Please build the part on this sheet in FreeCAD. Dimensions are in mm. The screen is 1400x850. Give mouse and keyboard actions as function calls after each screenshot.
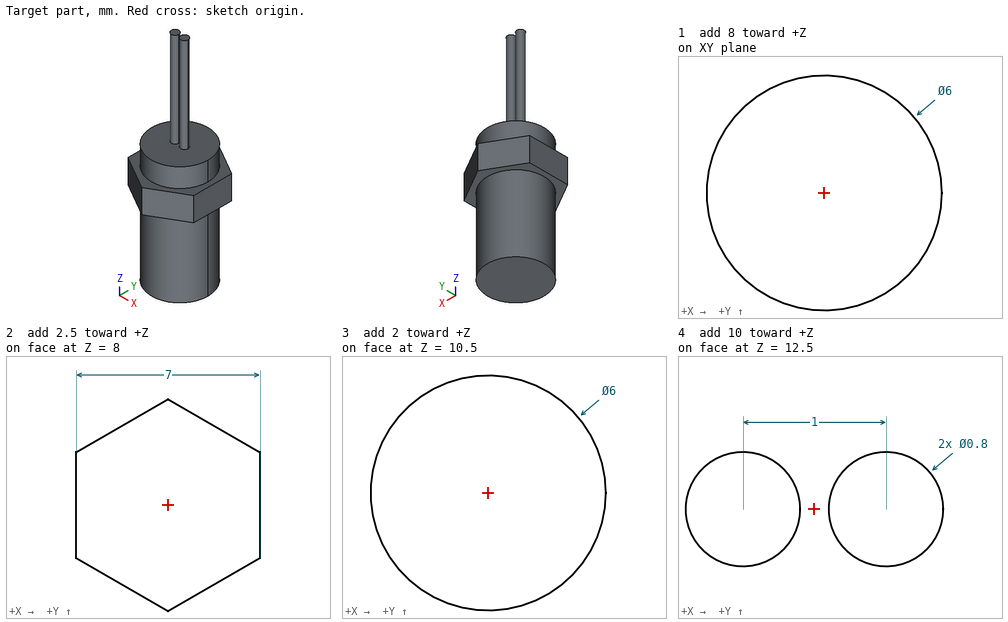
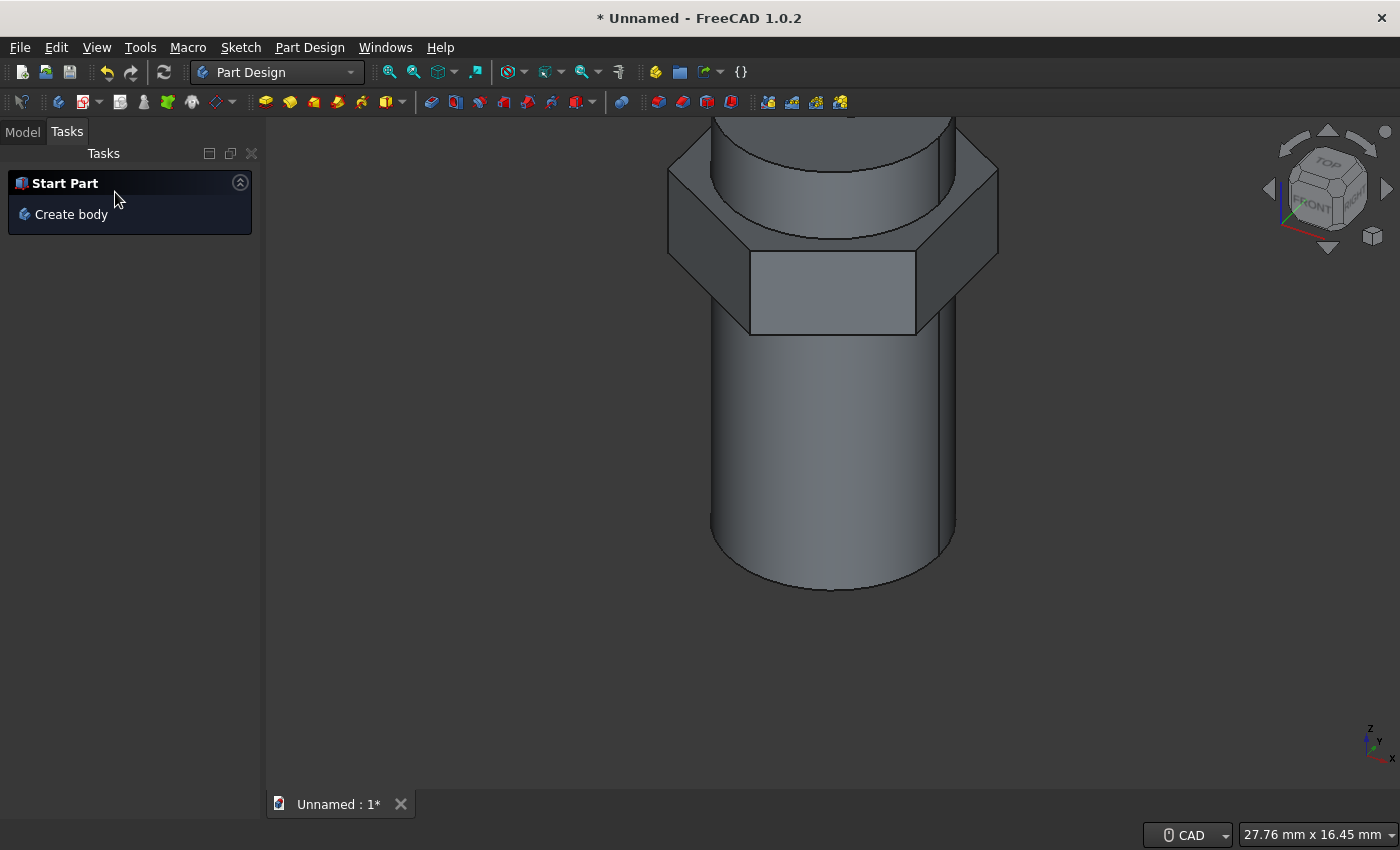
key(0)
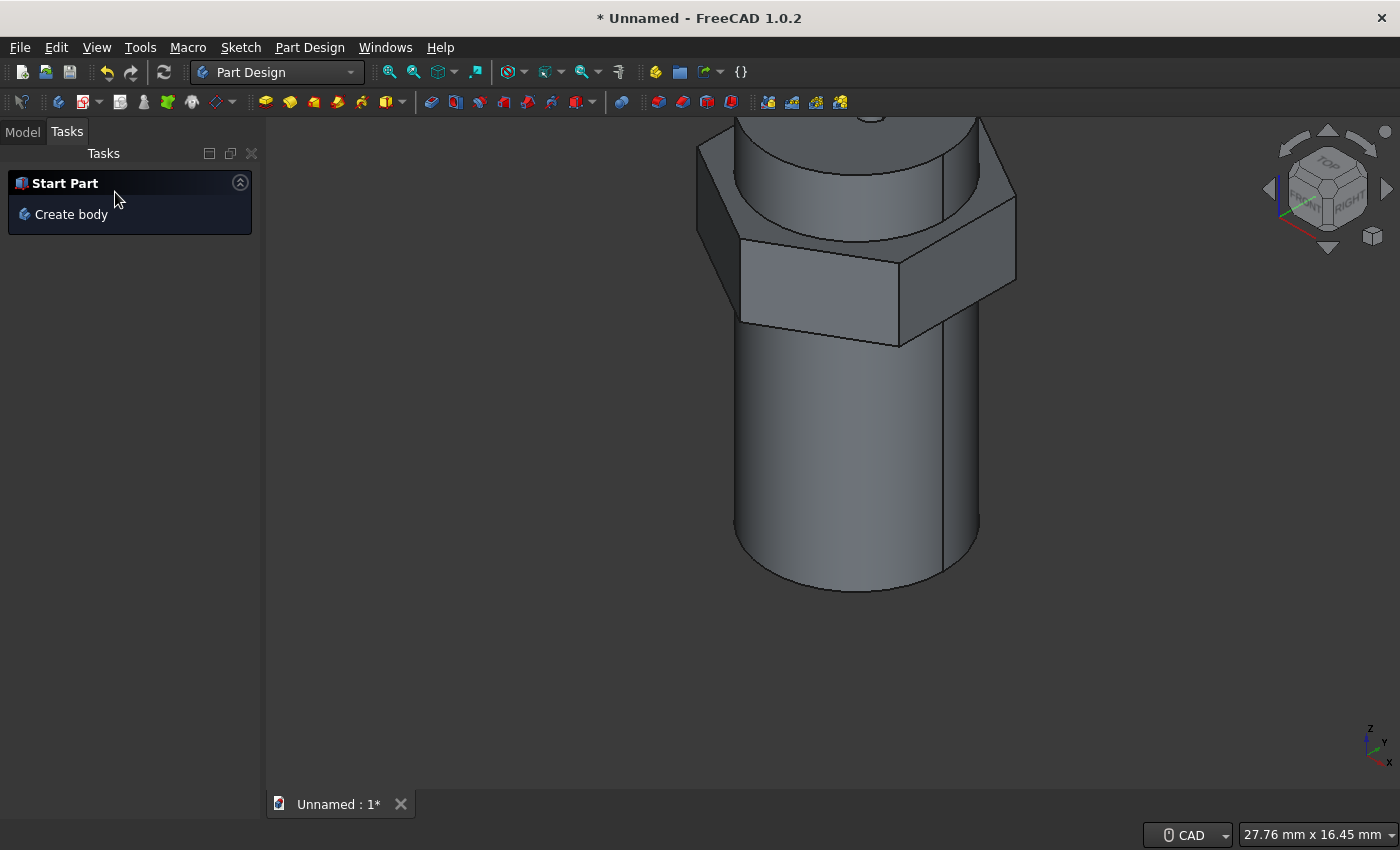
click(390, 72)